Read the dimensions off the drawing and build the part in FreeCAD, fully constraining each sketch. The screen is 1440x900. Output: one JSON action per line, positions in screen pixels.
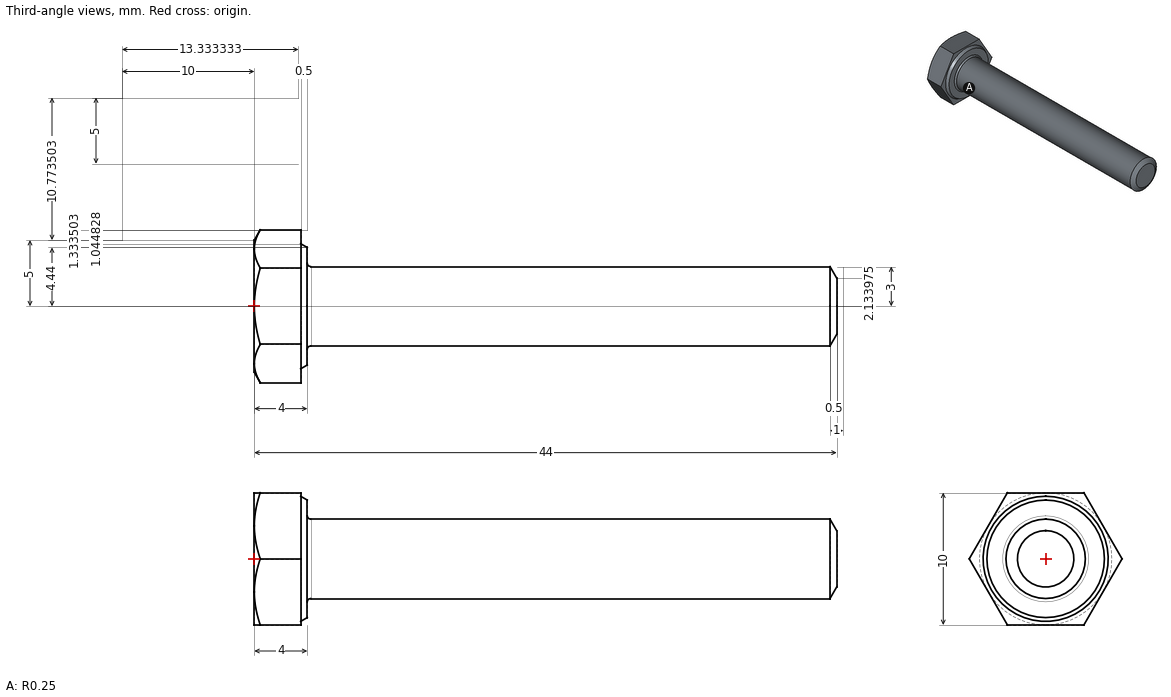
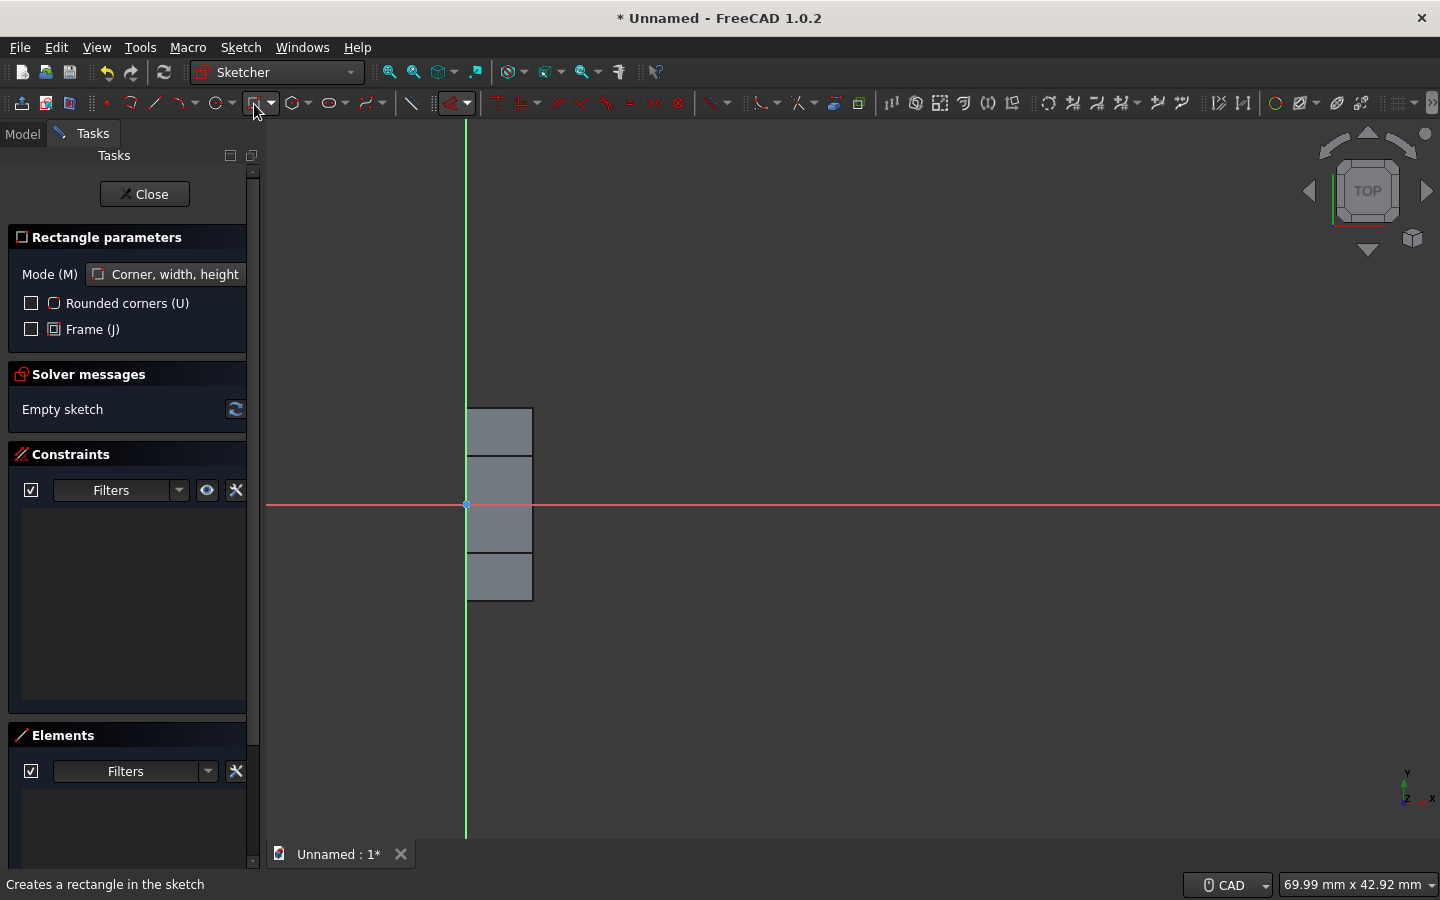
{"action": "left_click", "coordinate": [466, 505]}
{"action": "left_click", "coordinate": [1204, 454]}
{"action": "key", "text": "Escape"}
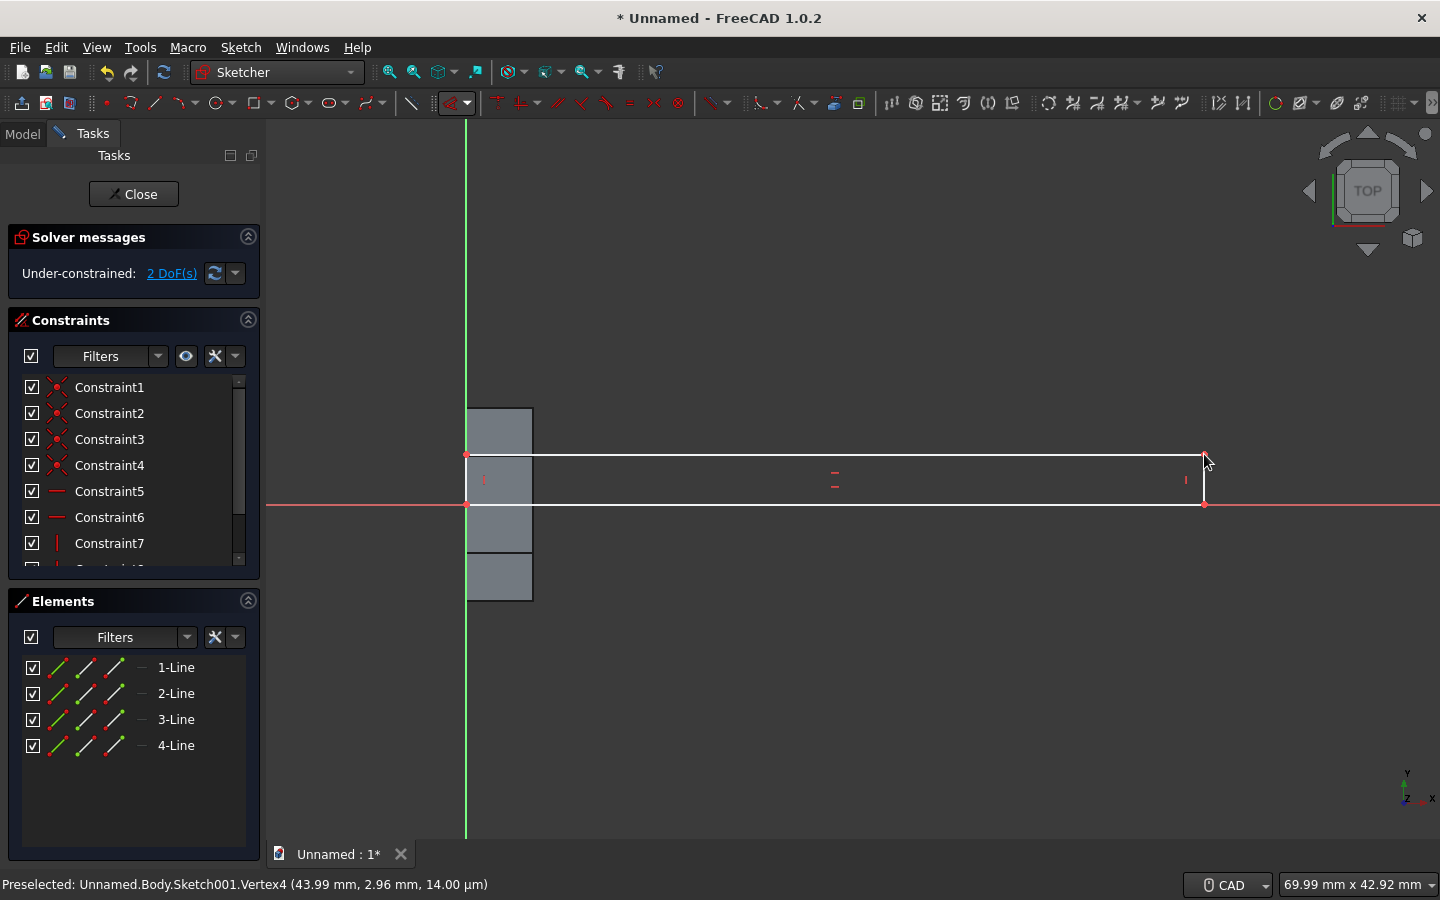
{"action": "left_click", "coordinate": [1204, 490]}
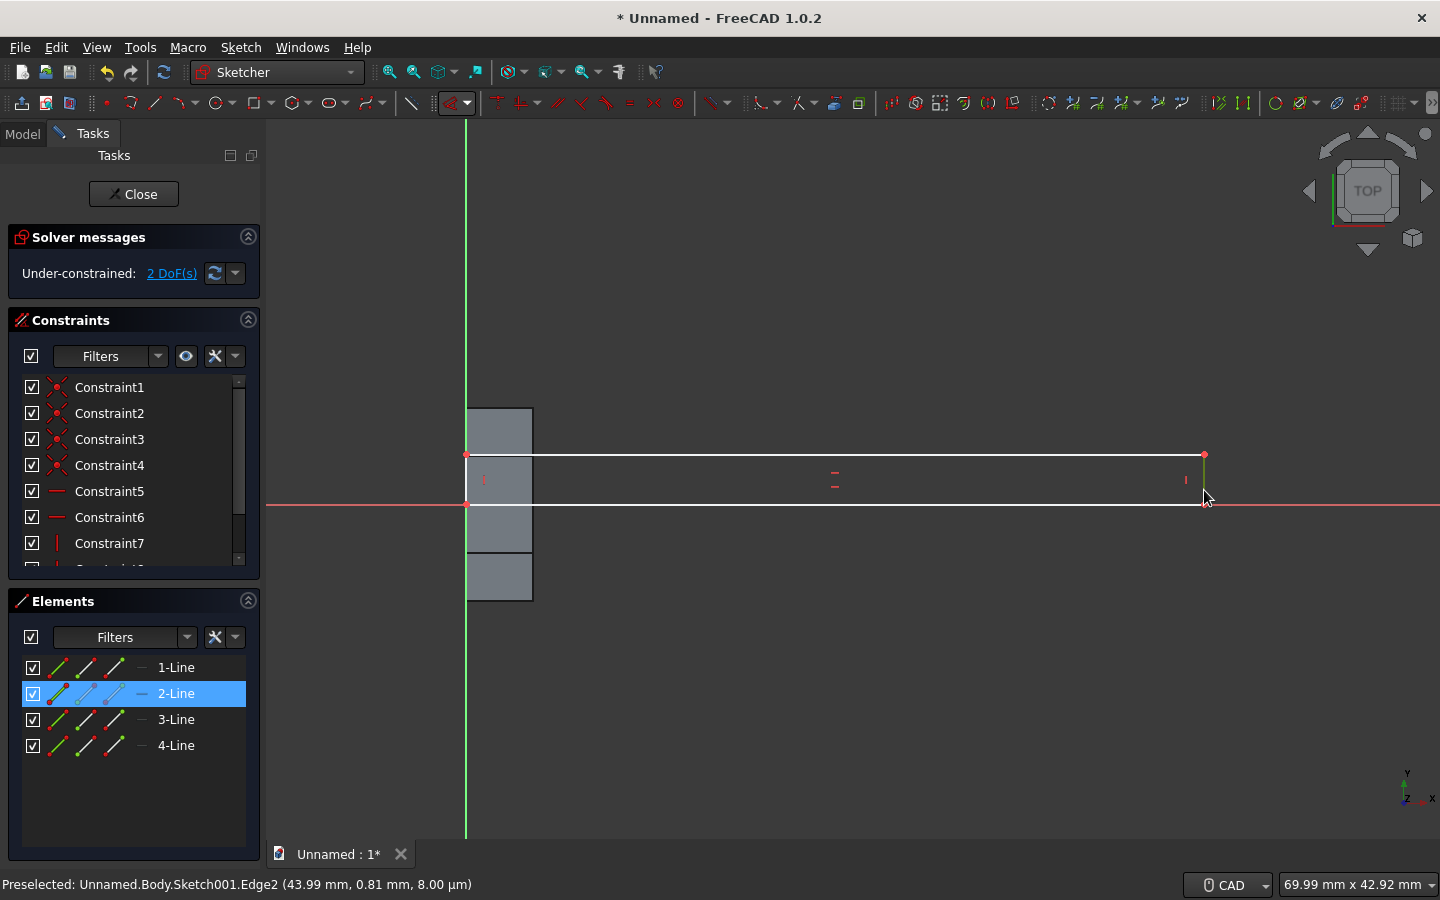
{"action": "key", "text": "i"}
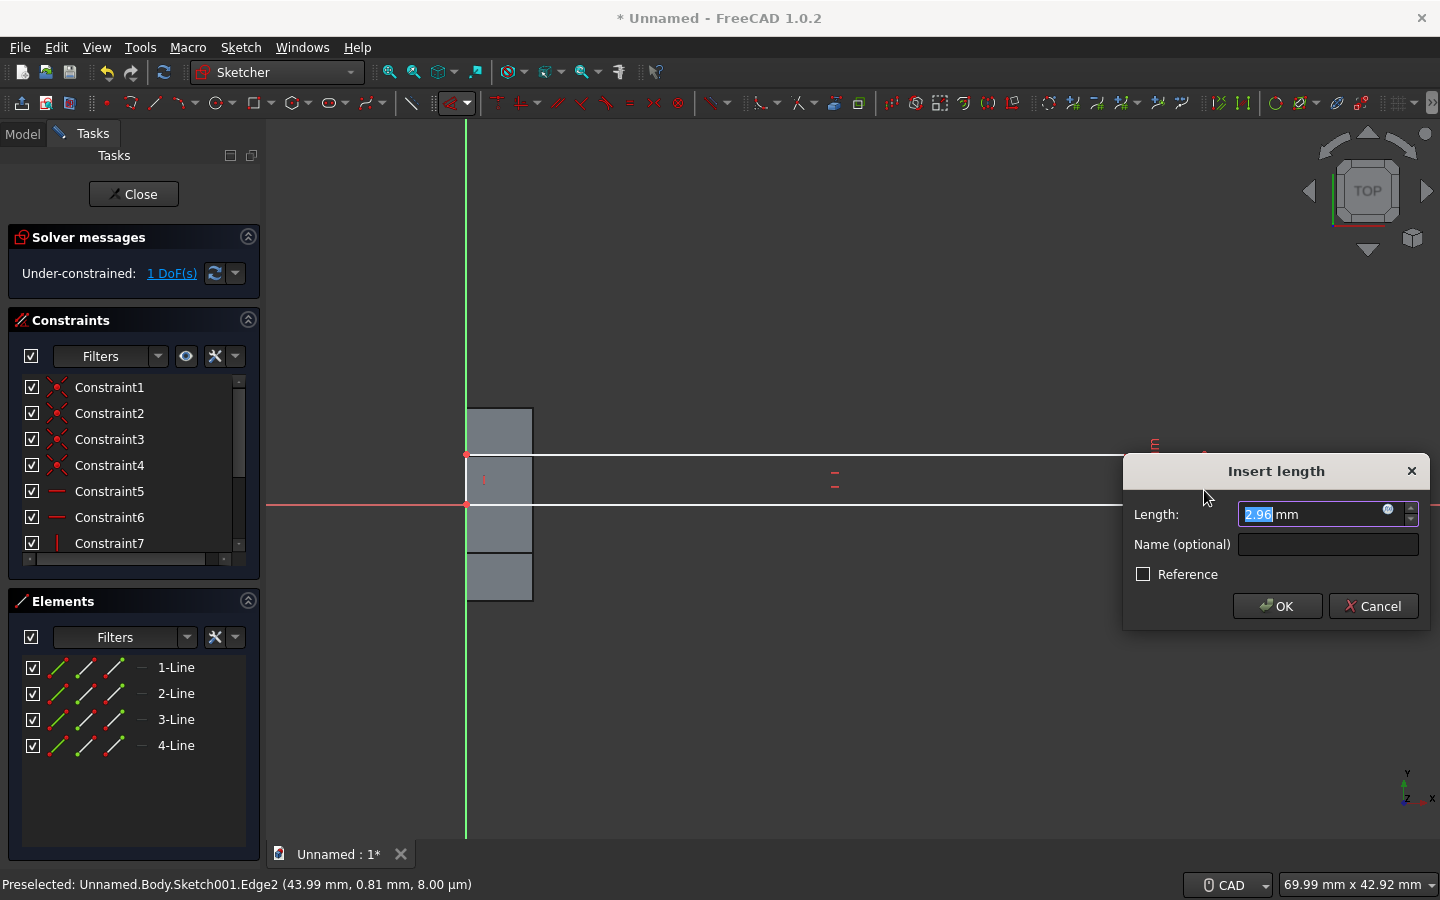
{"action": "type", "text": "3"}
{"action": "key", "text": "Return"}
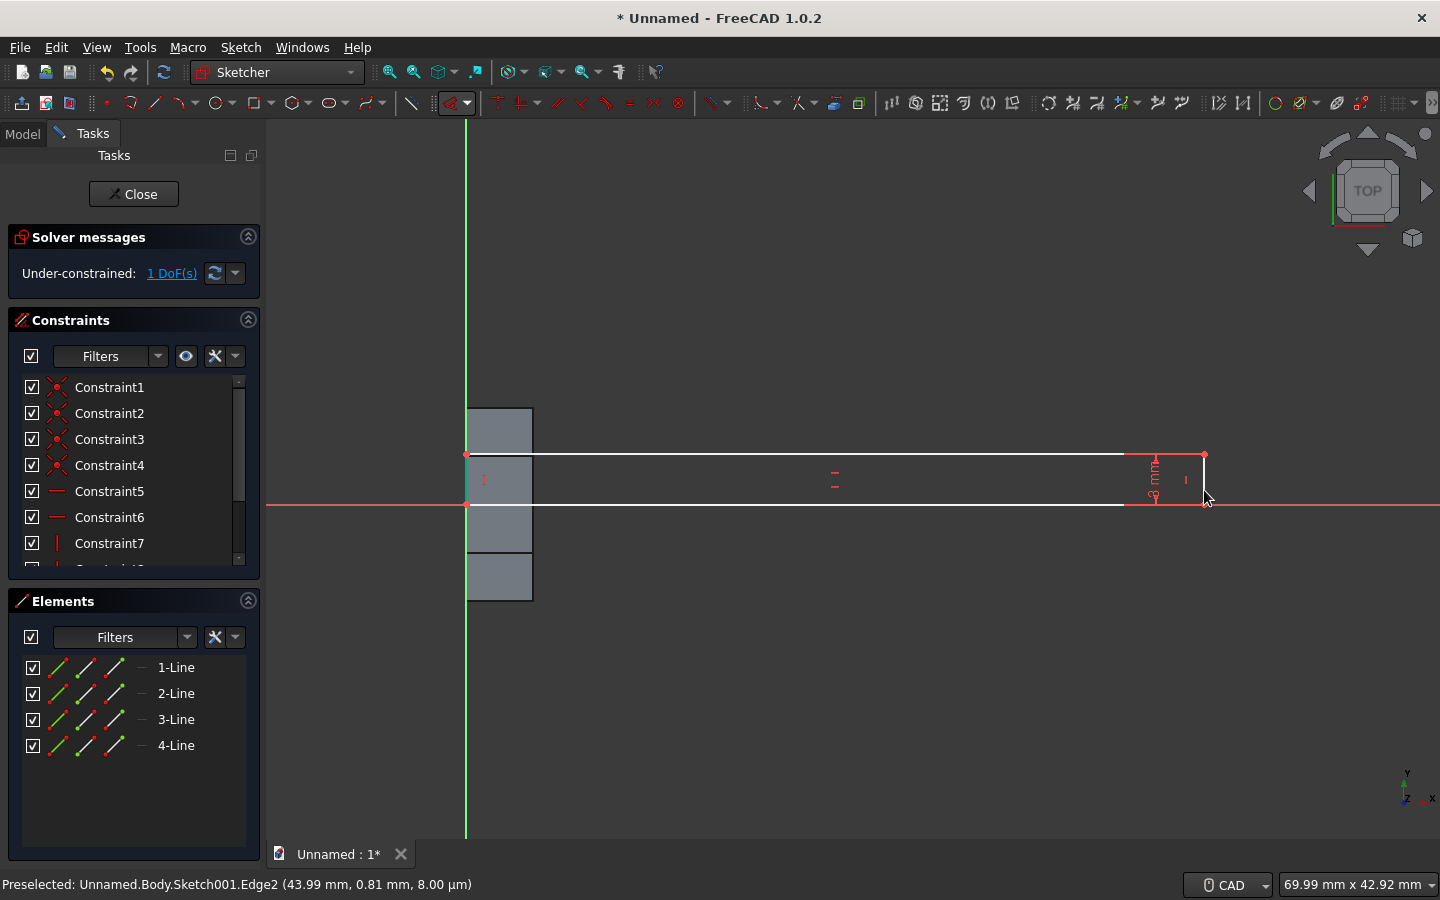
{"action": "left_click", "coordinate": [687, 505]}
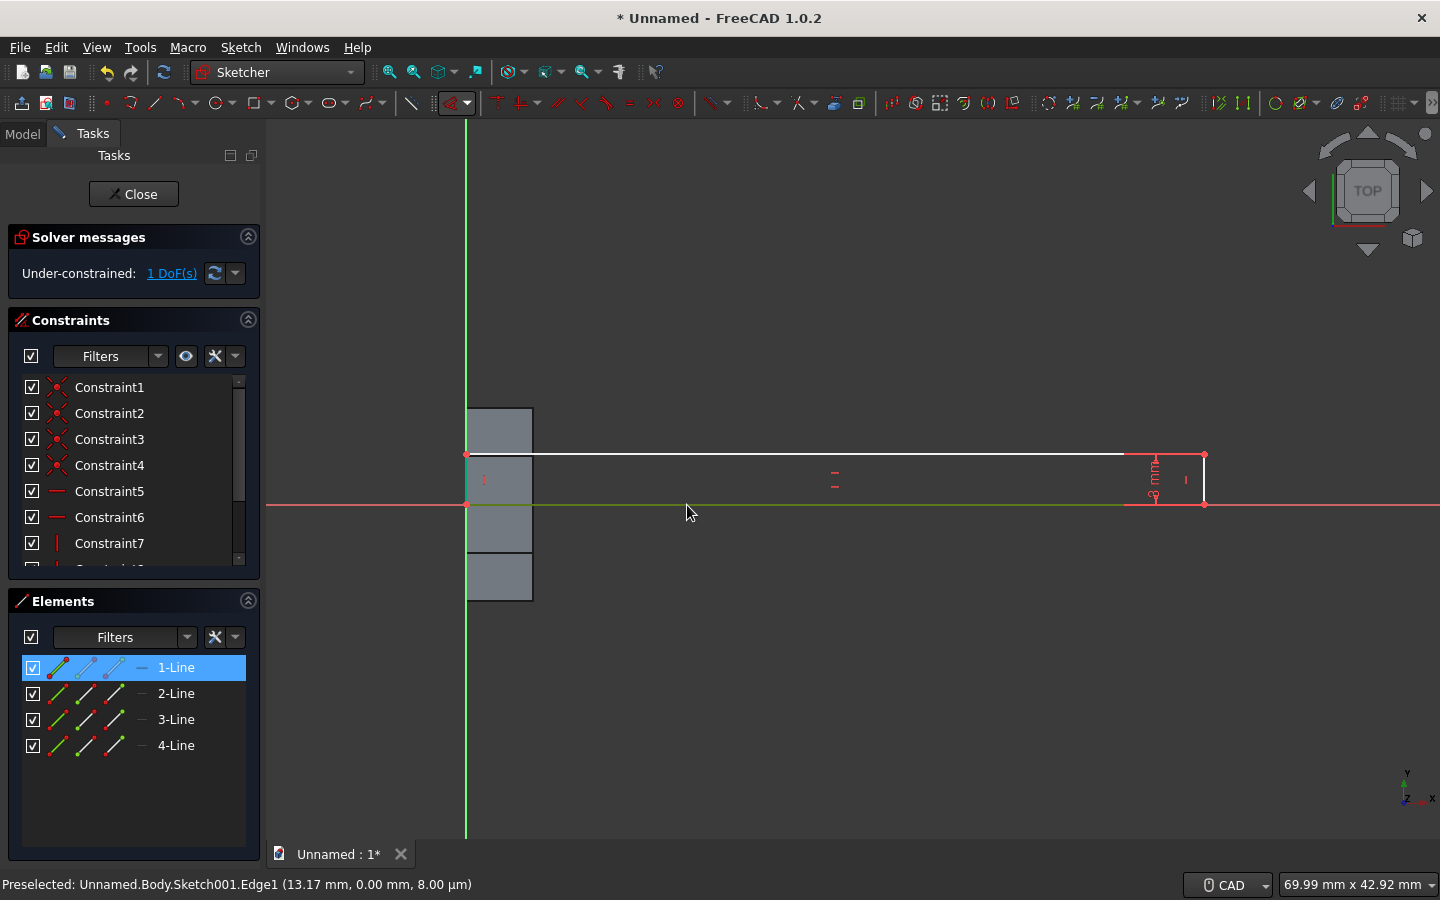
{"action": "left_click", "coordinate": [470, 104]}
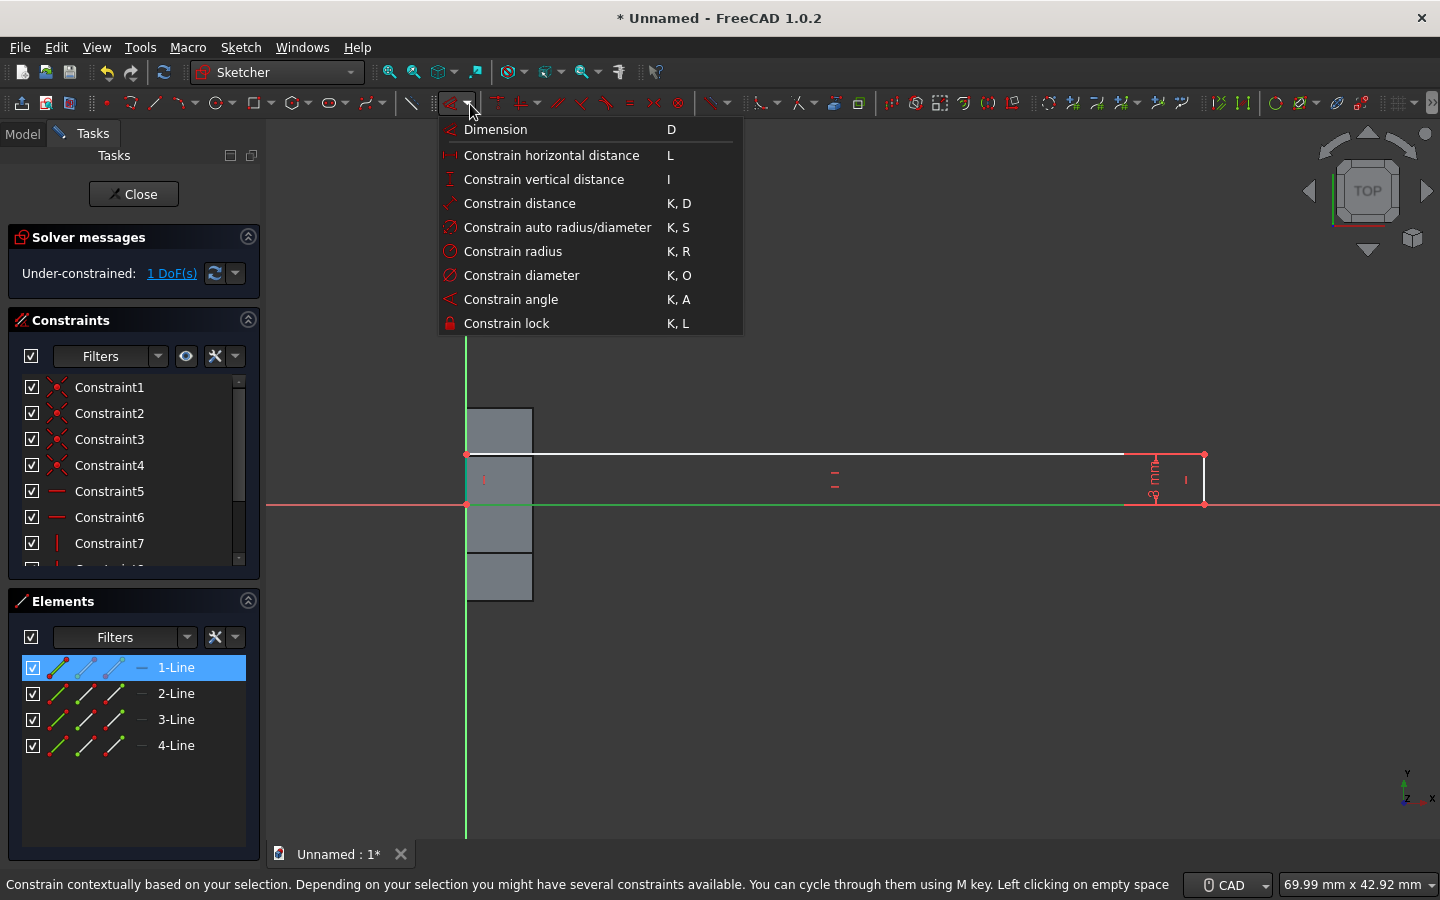
{"action": "left_click", "coordinate": [591, 155]}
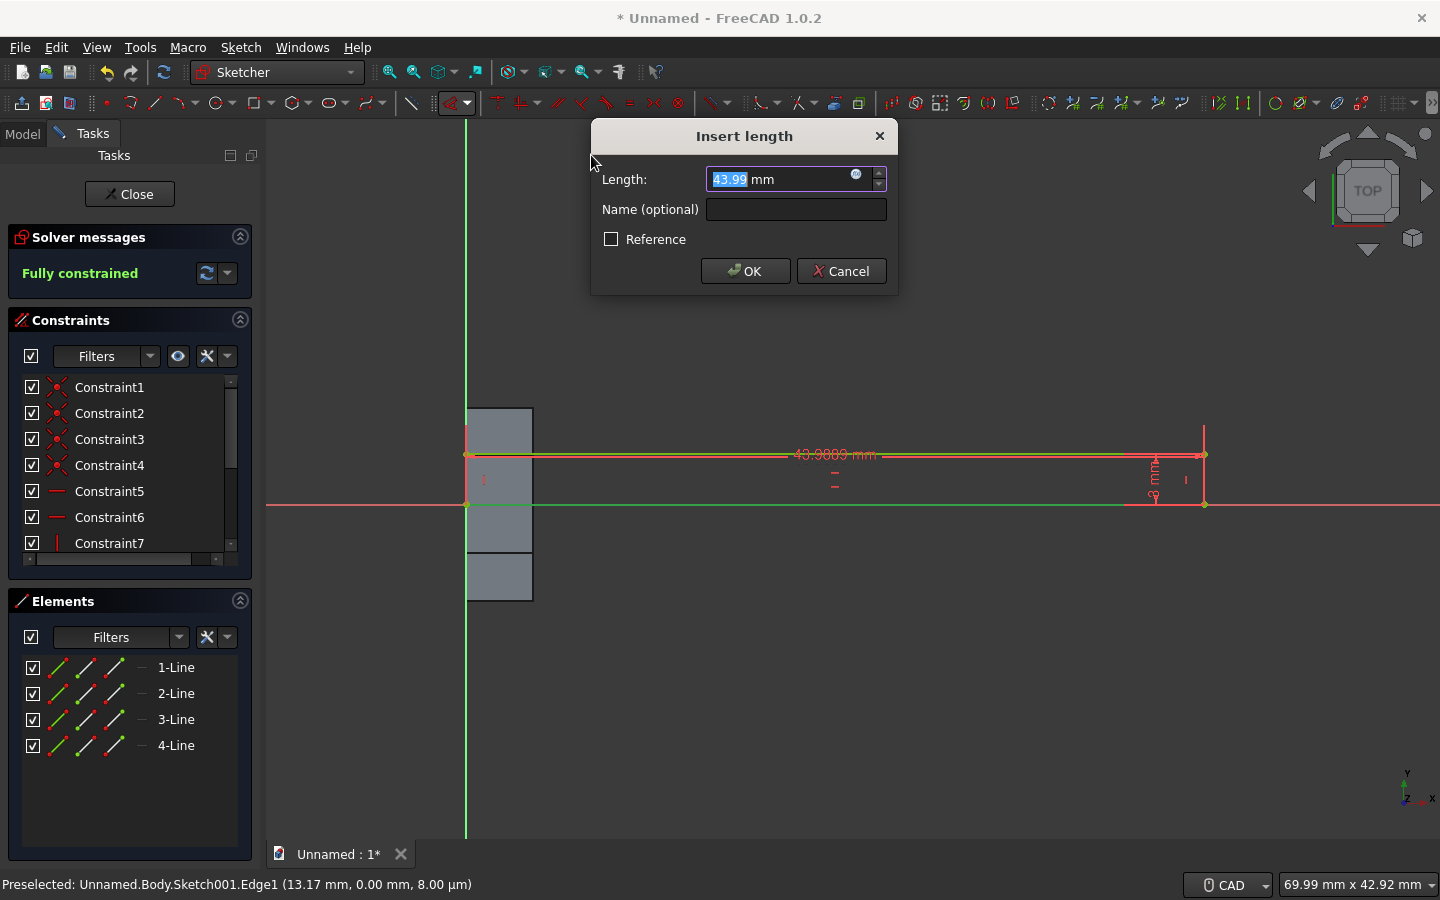
{"action": "type", "text": "44"}
{"action": "key", "text": "Return"}